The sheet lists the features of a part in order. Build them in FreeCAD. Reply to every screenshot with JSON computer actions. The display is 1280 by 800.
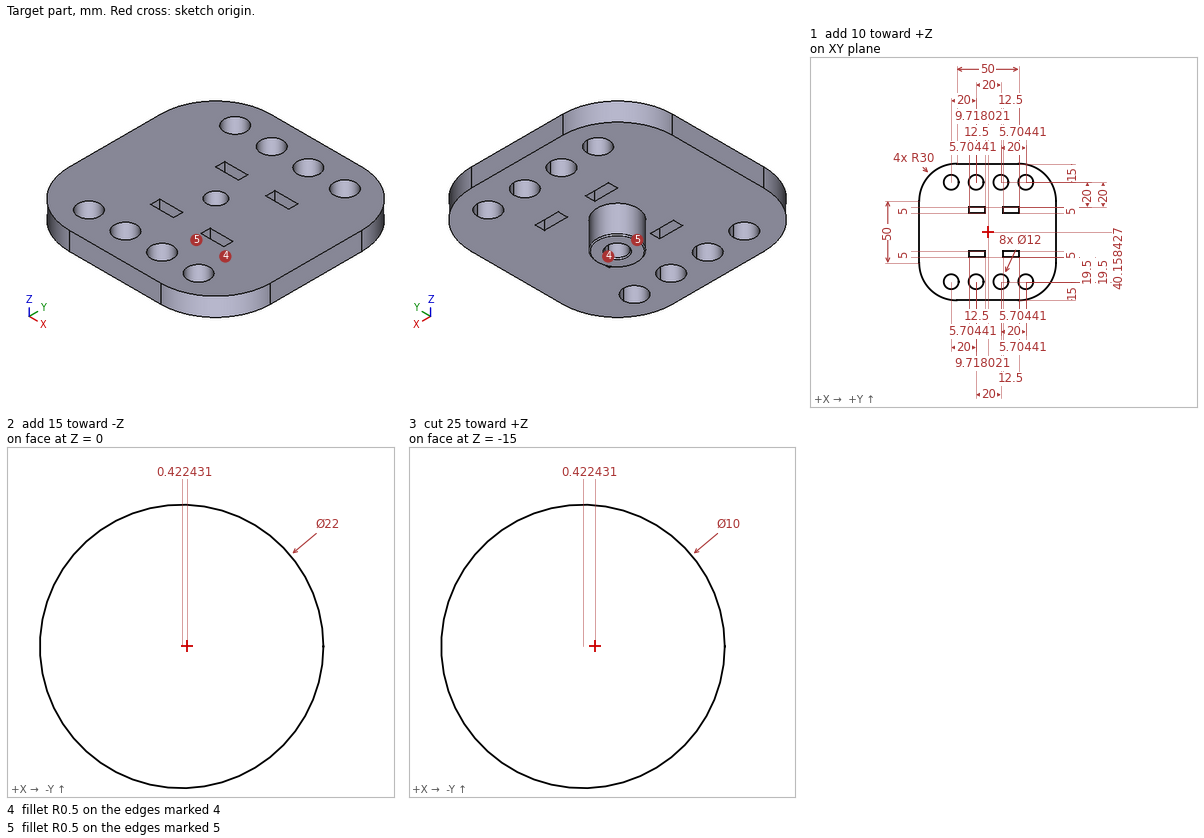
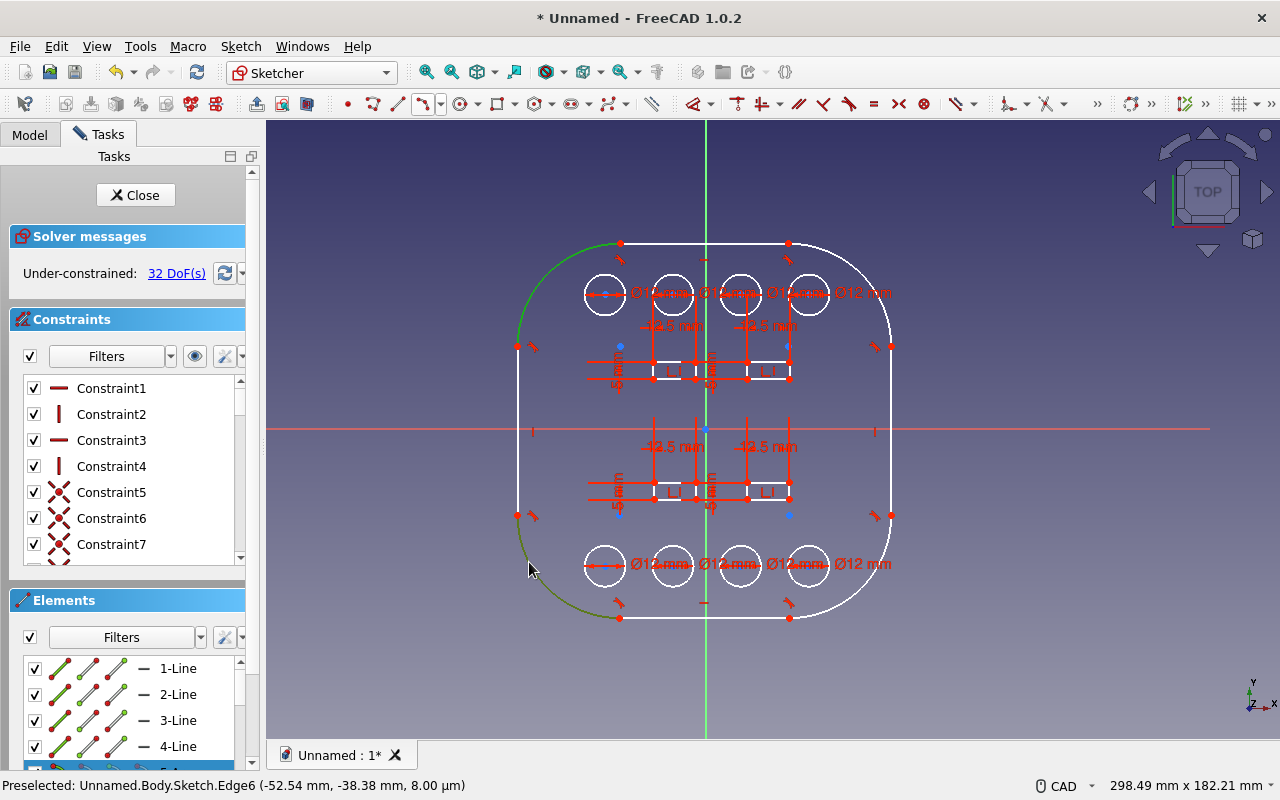
{"action": "left_click", "coordinate": [835, 607]}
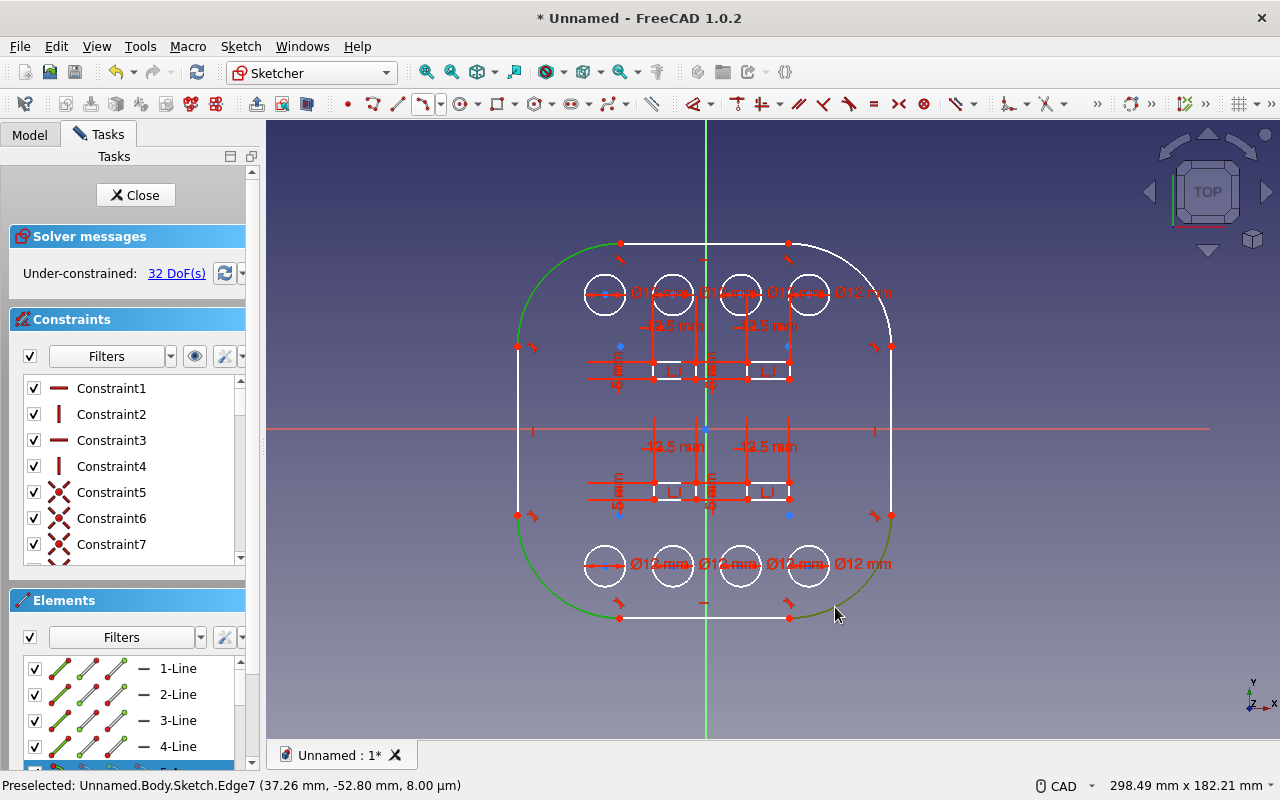
{"action": "left_click", "coordinate": [880, 300]}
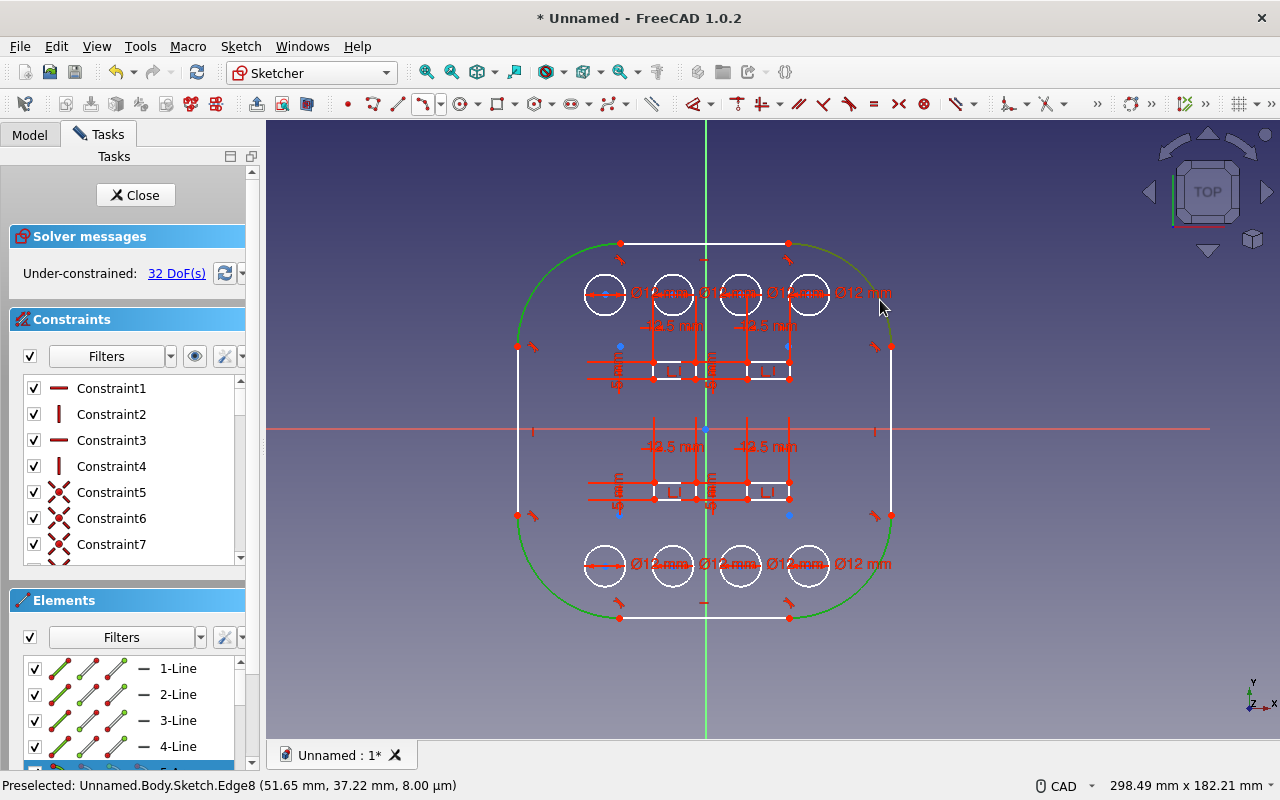
{"action": "left_click", "coordinate": [874, 104]}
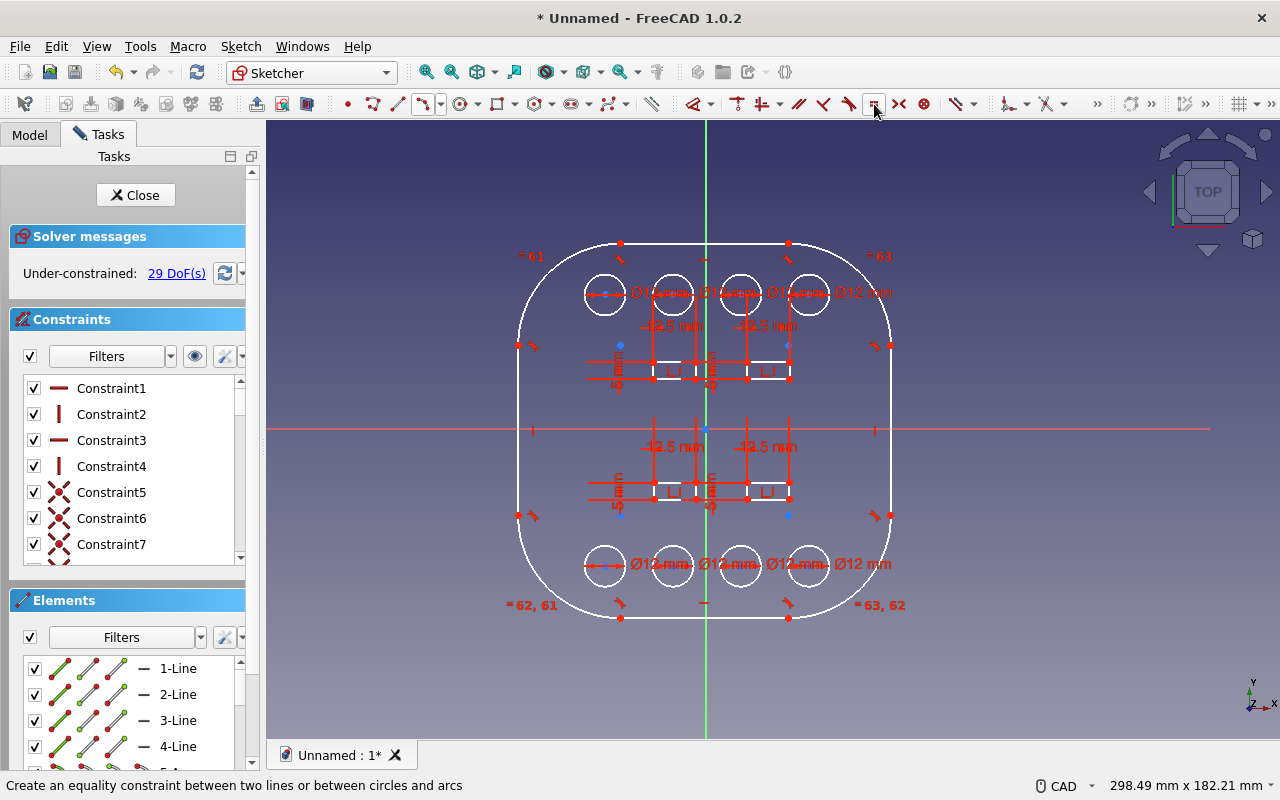
{"action": "left_click", "coordinate": [809, 566]}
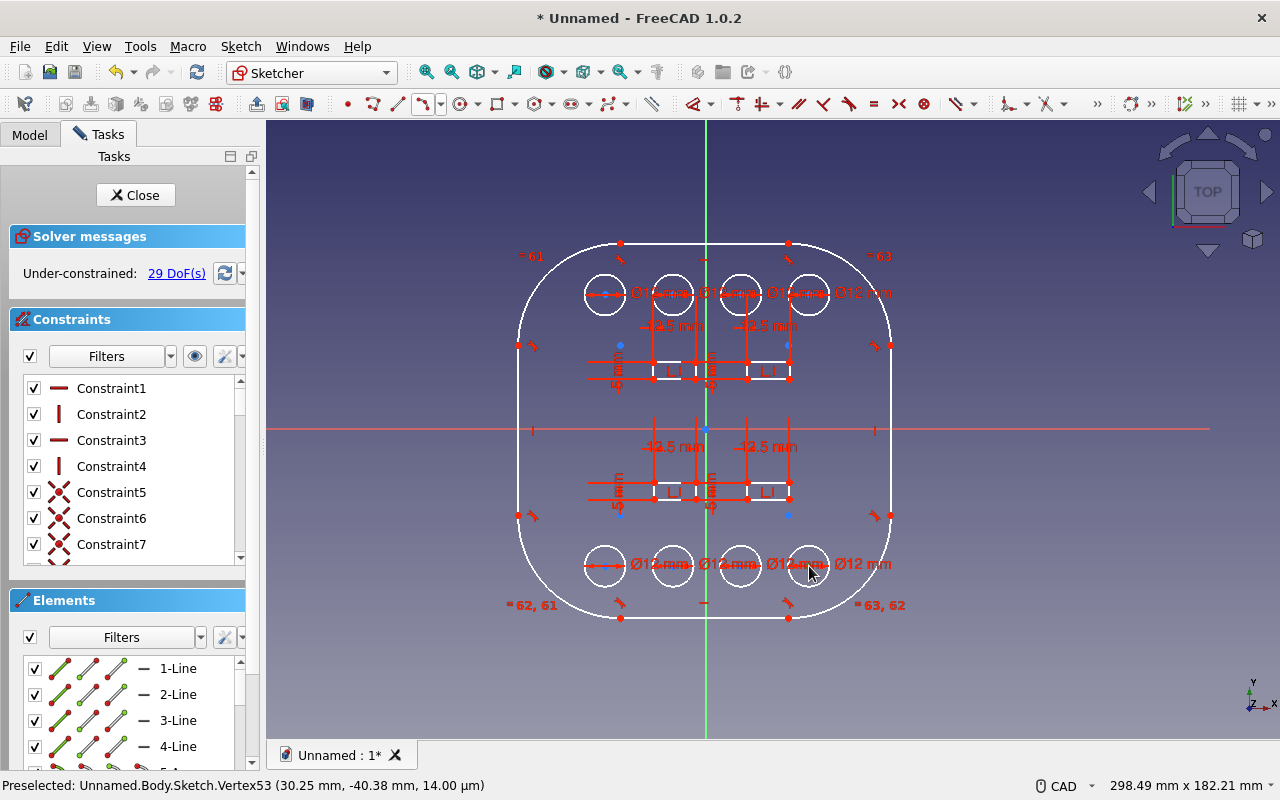
{"action": "left_click", "coordinate": [741, 566]}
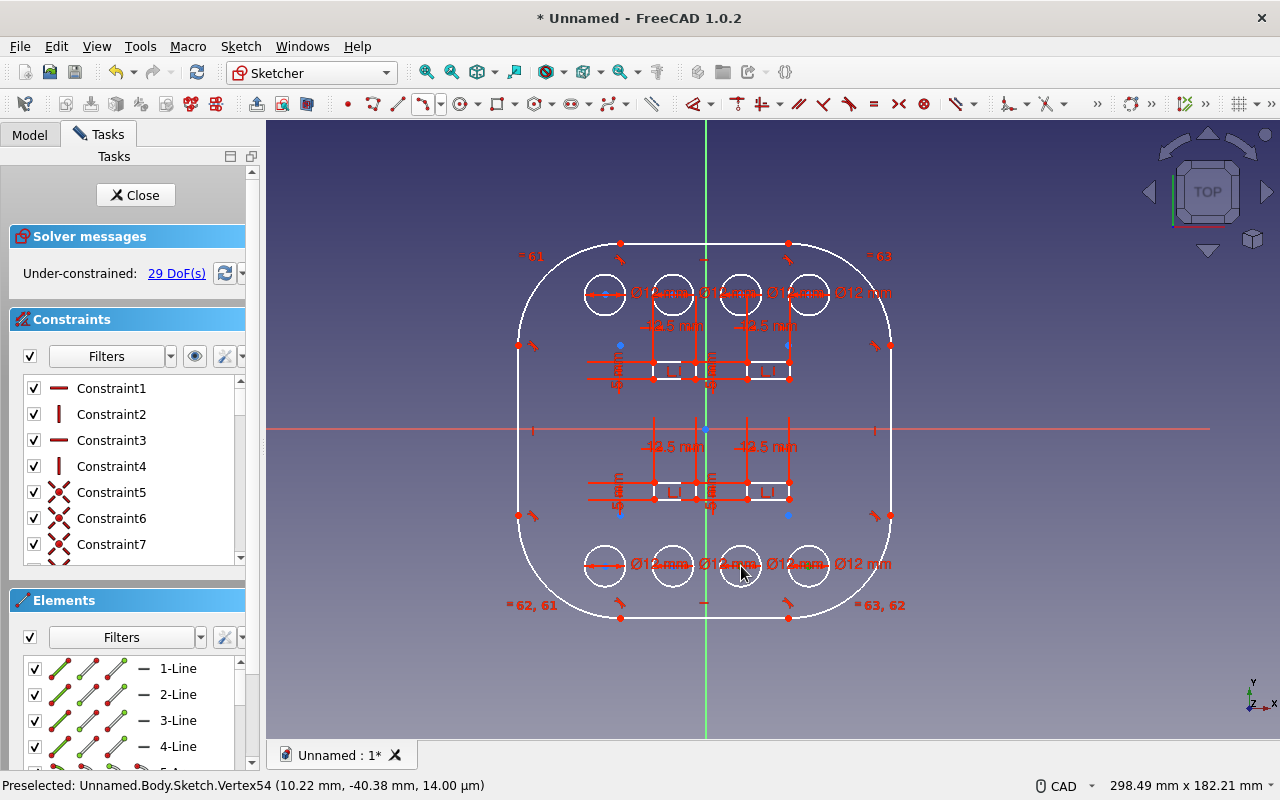
{"action": "left_click", "coordinate": [780, 104]}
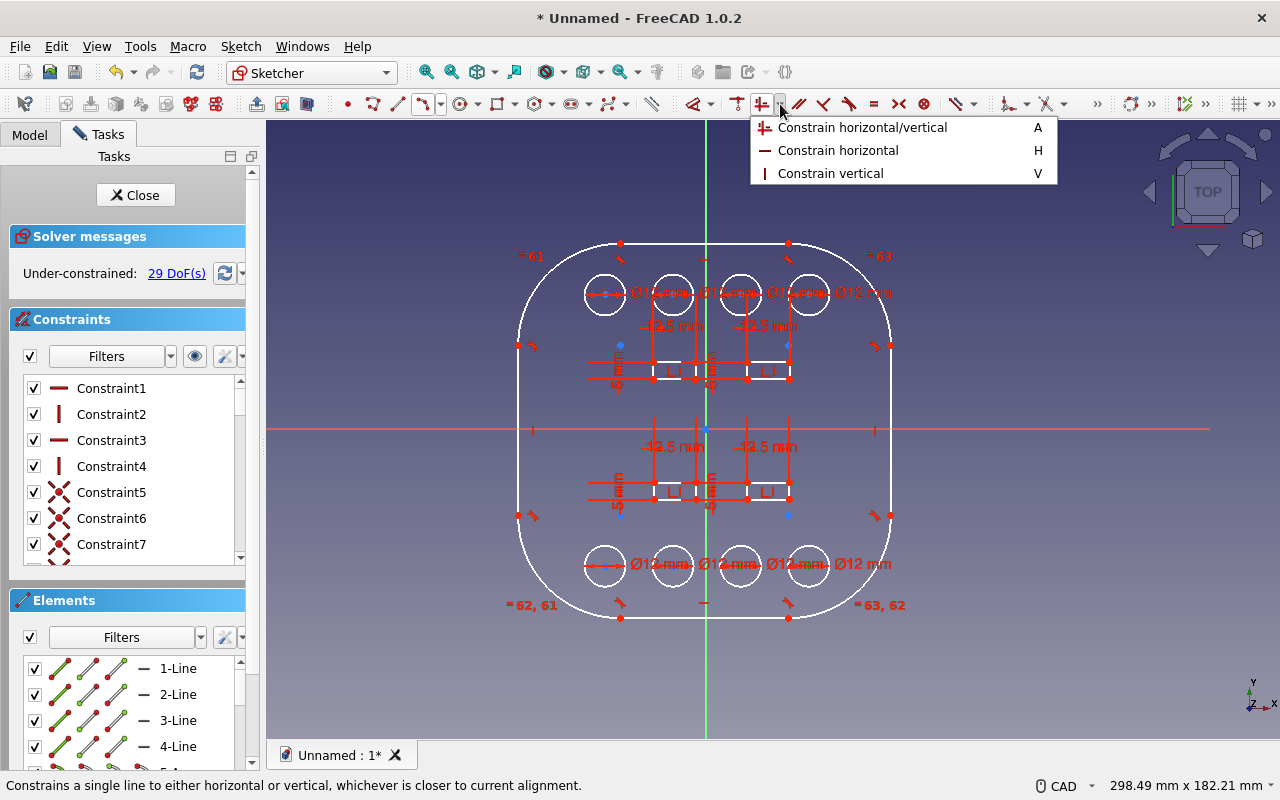
{"action": "left_click", "coordinate": [904, 150]}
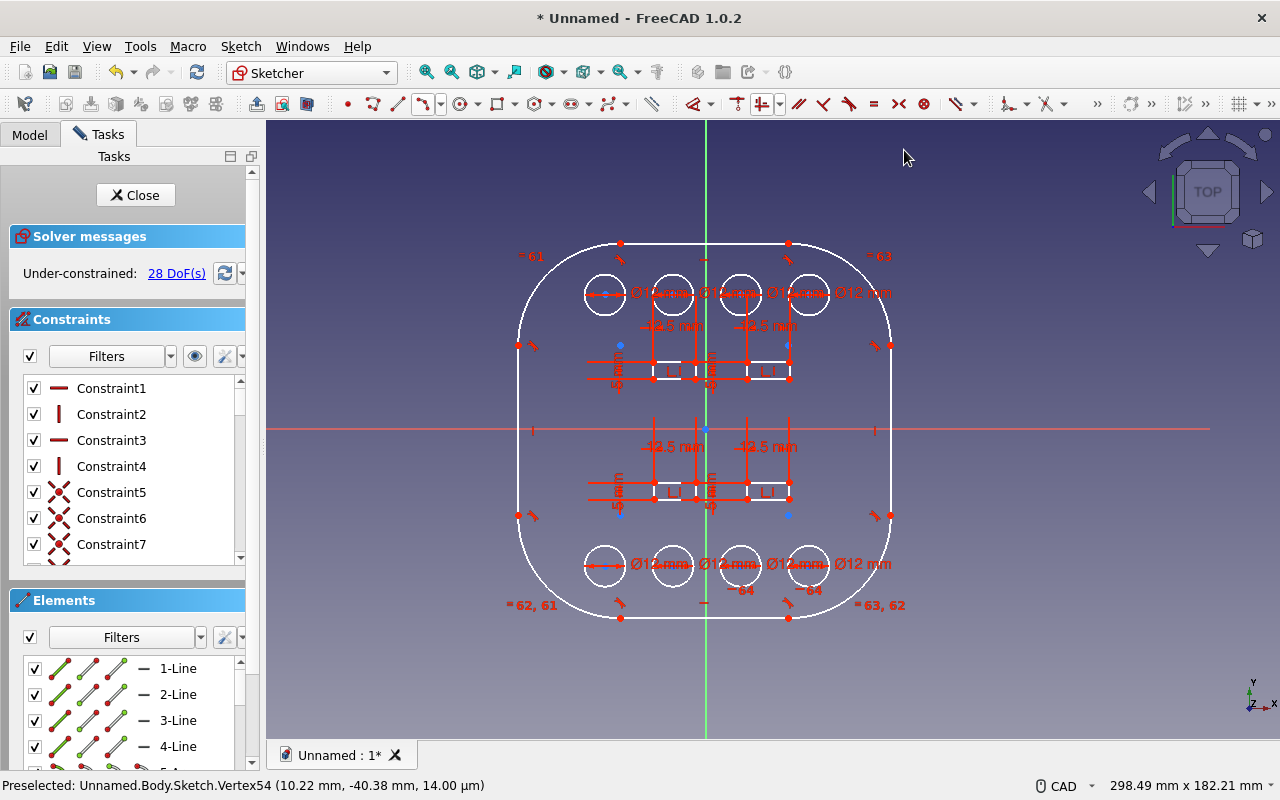
{"action": "left_click", "coordinate": [741, 566]}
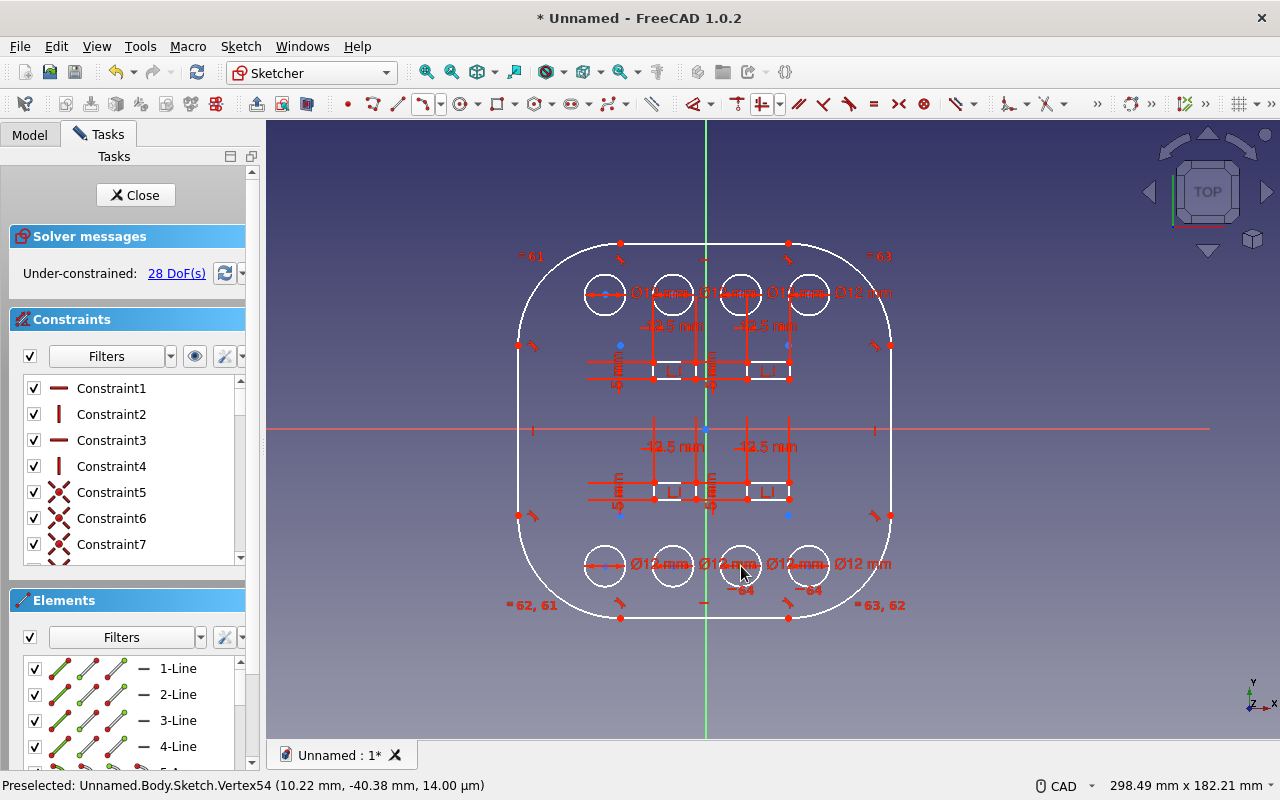
{"action": "left_click", "coordinate": [673, 566]}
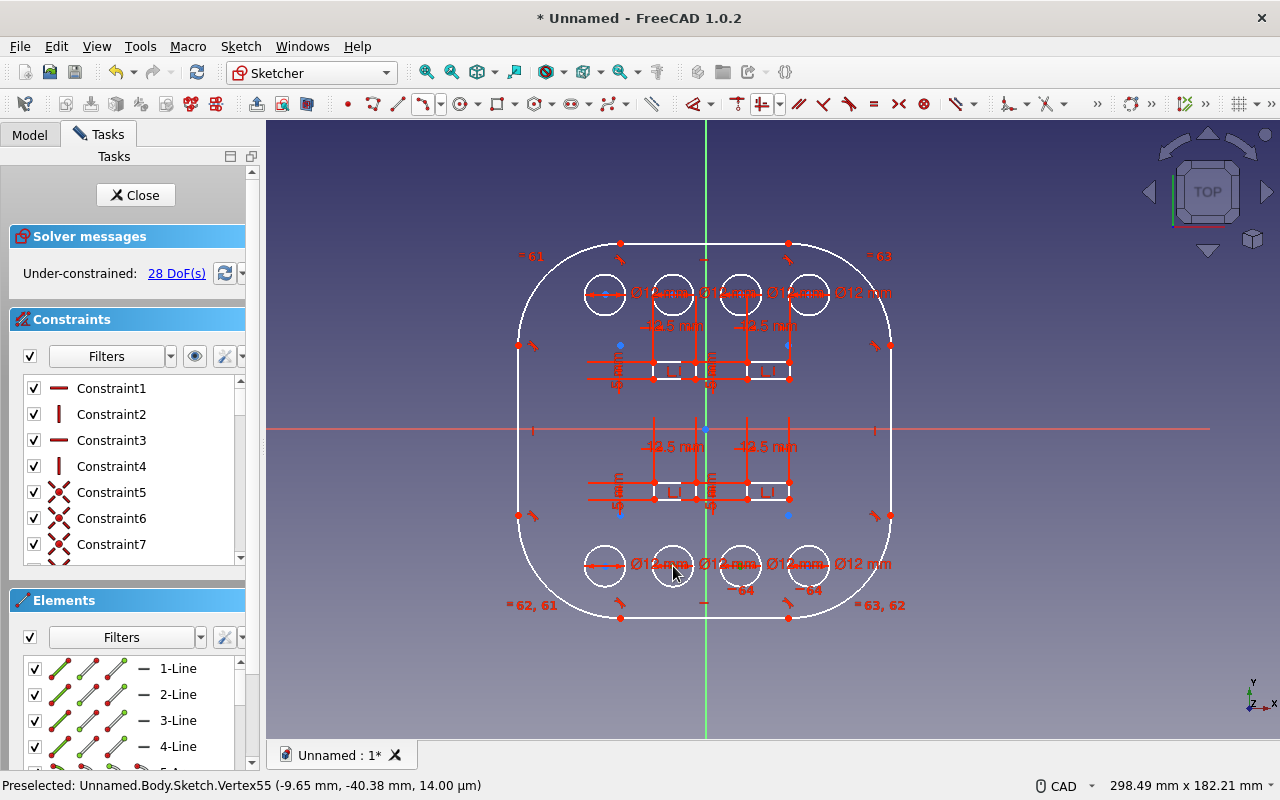
{"action": "key", "text": "h"}